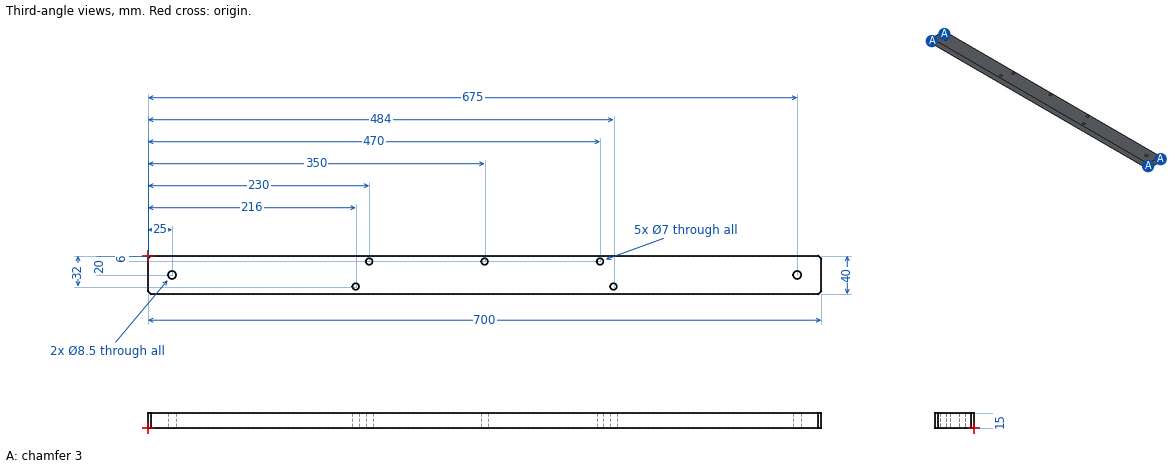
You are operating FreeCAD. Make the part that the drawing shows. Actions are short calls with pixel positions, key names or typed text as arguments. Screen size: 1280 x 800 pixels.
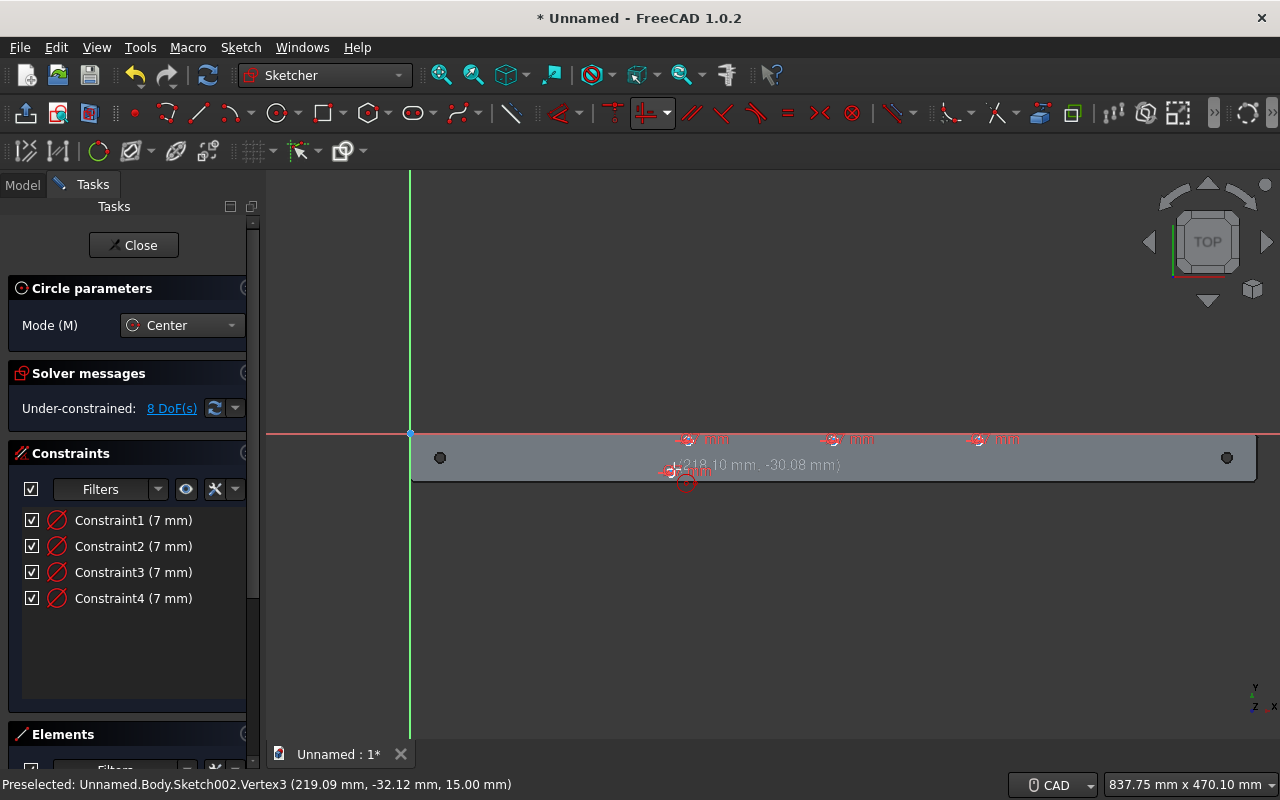
scroll(996, 472, up, 9)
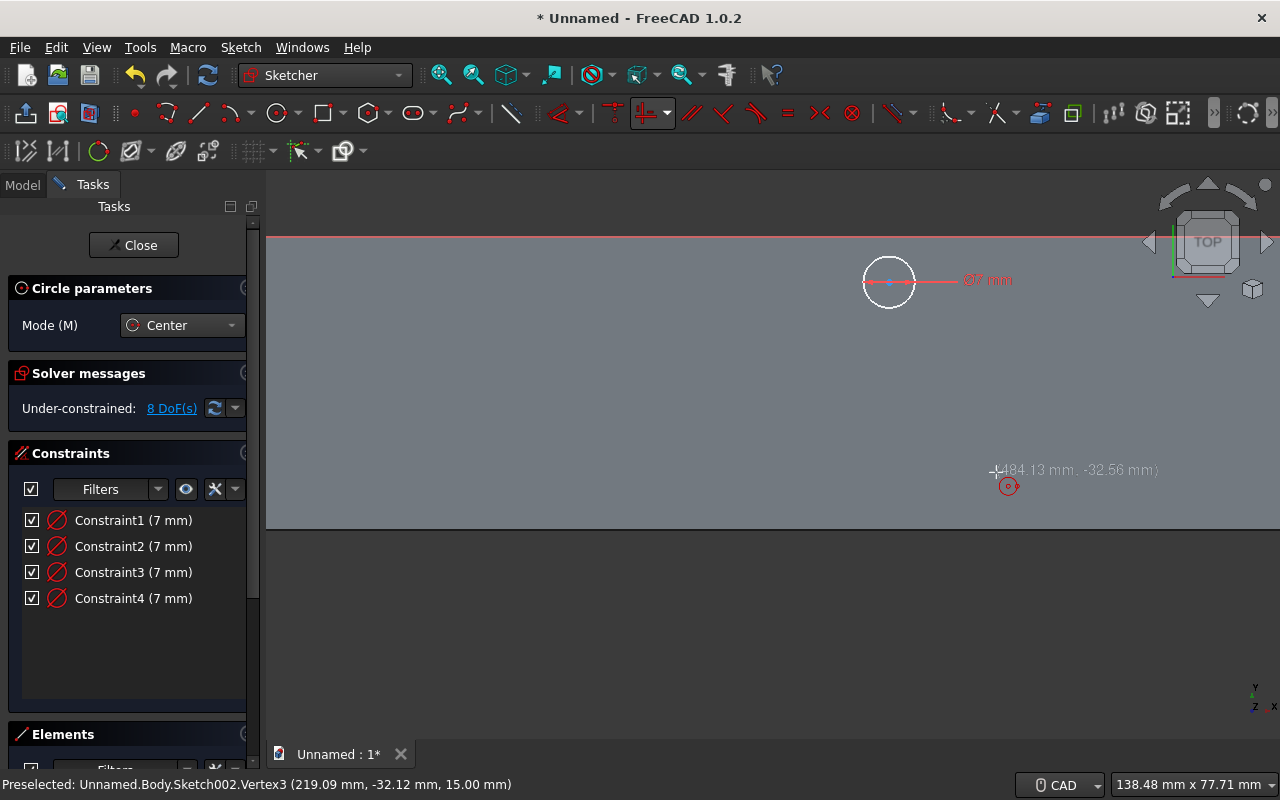
scroll(996, 472, down, 9)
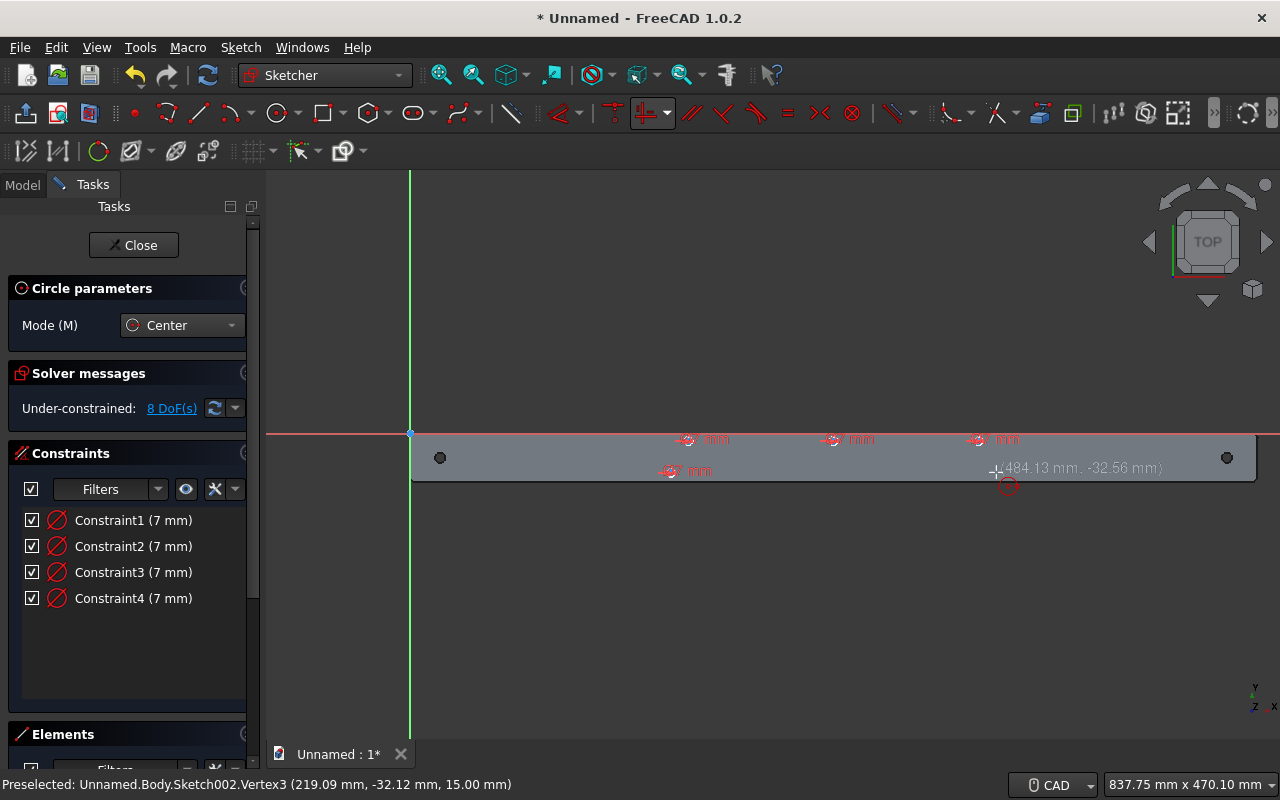
click(996, 472)
move(999, 469)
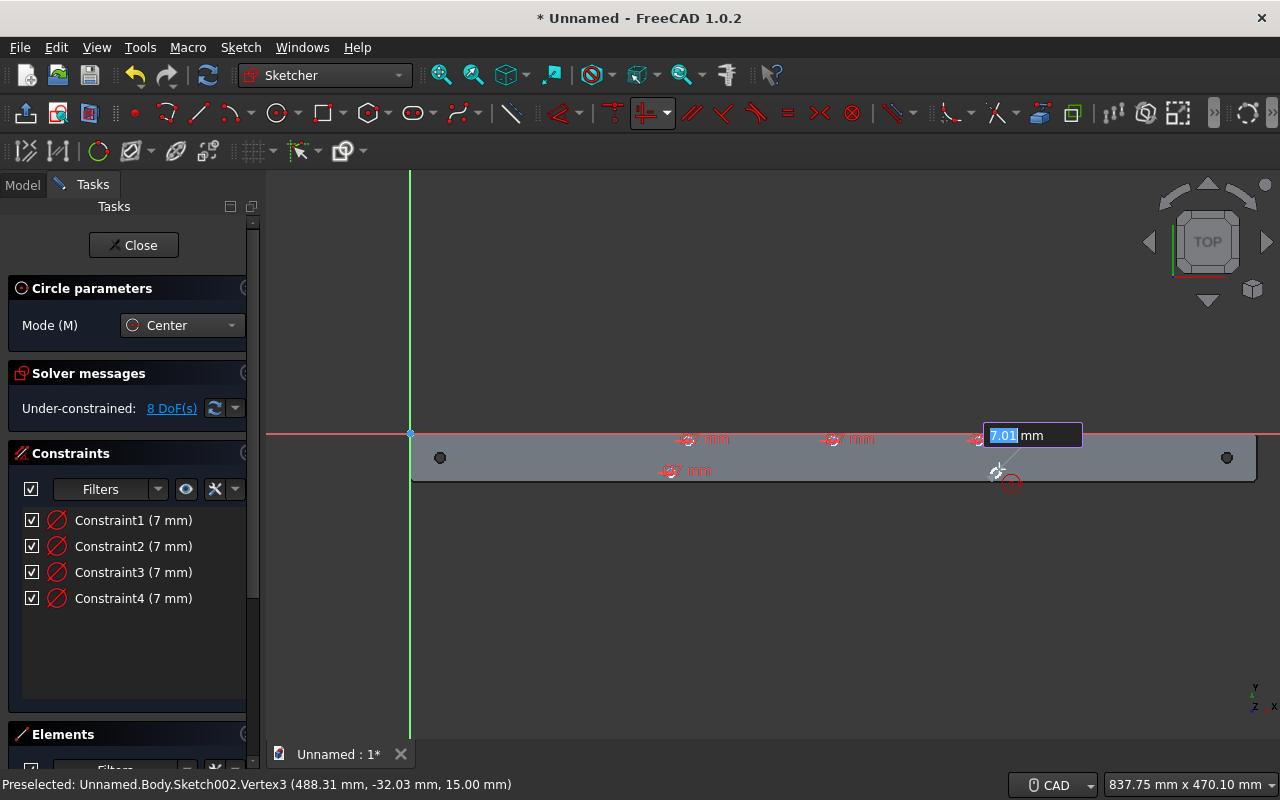
text(7)
key(Return)
key(Escape)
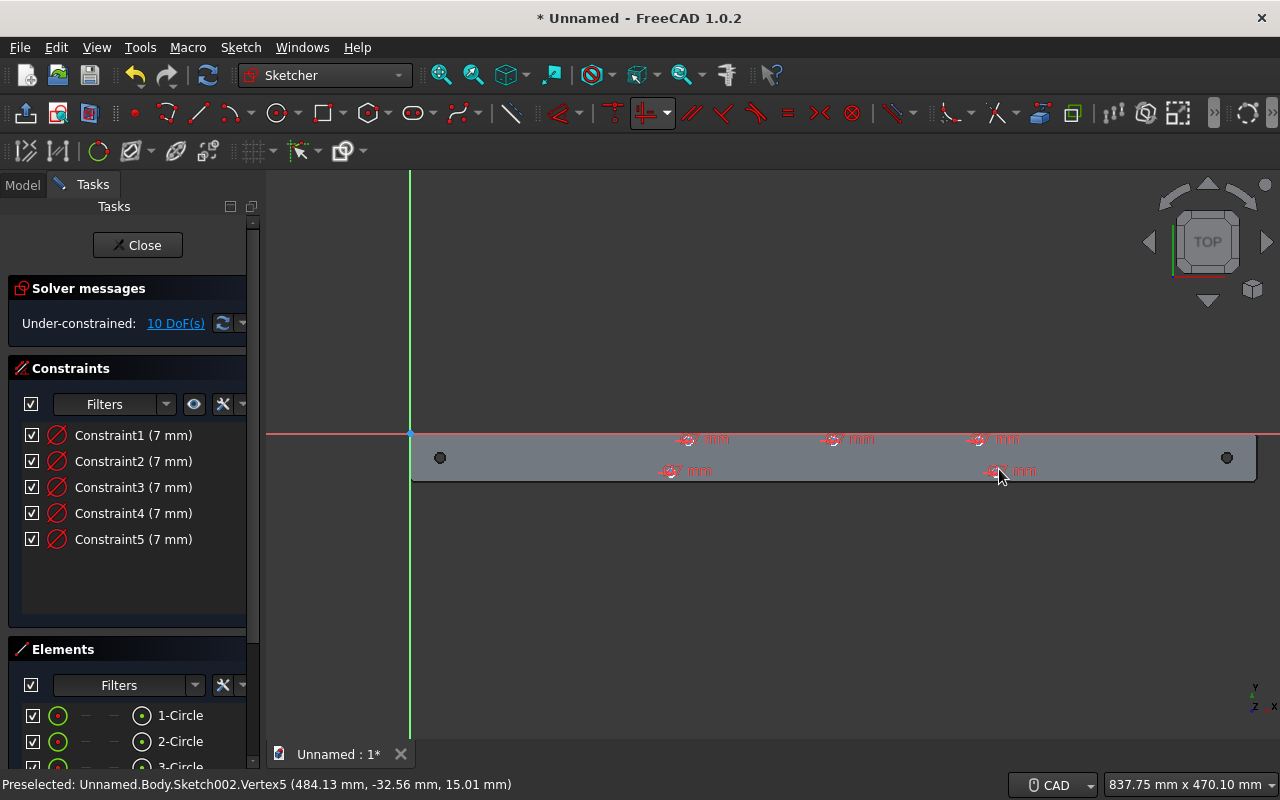
click(979, 441)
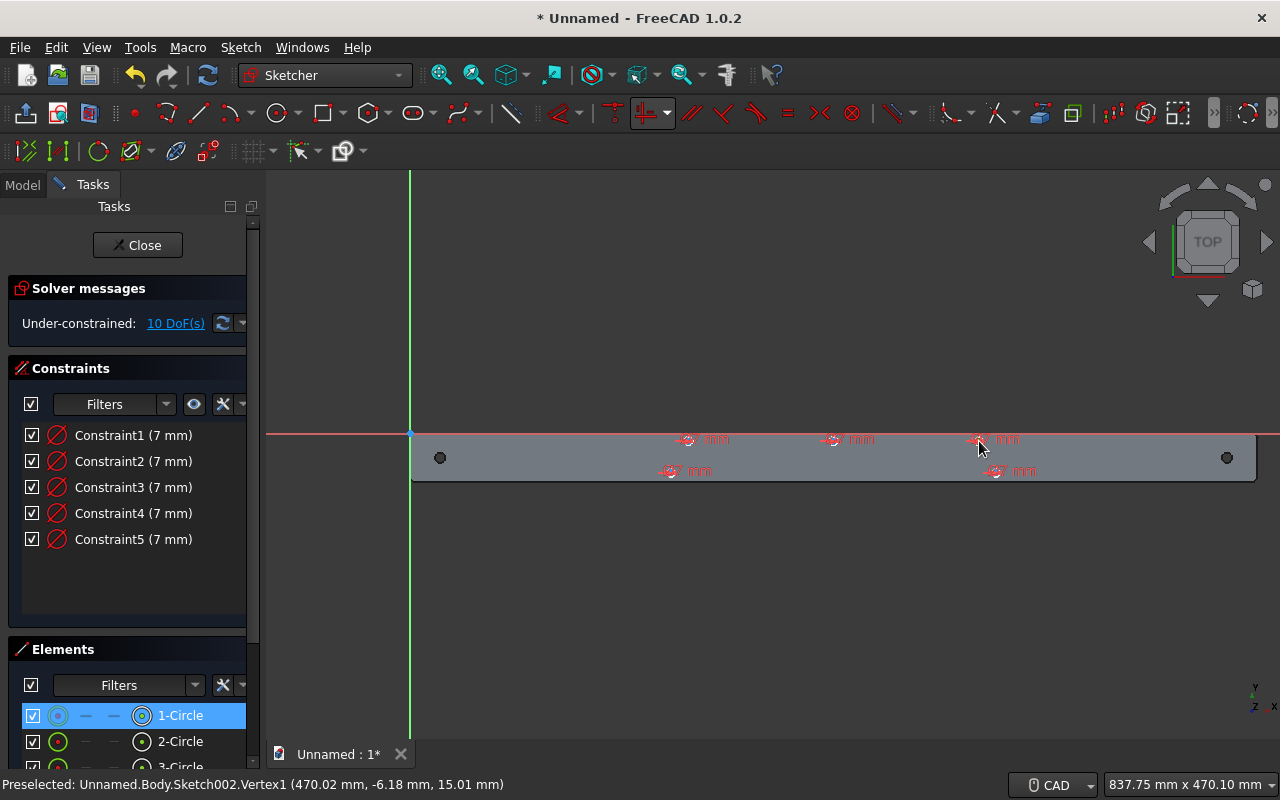
click(834, 441)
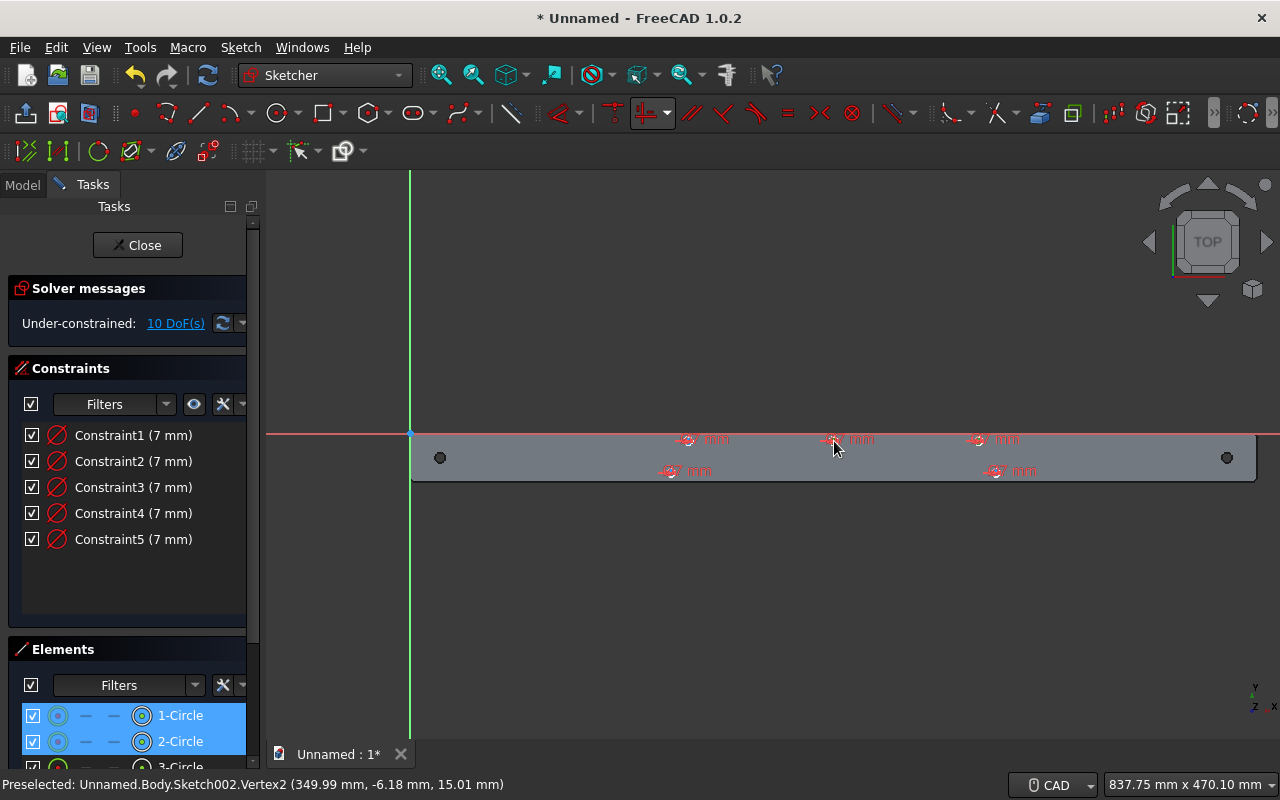
click(670, 114)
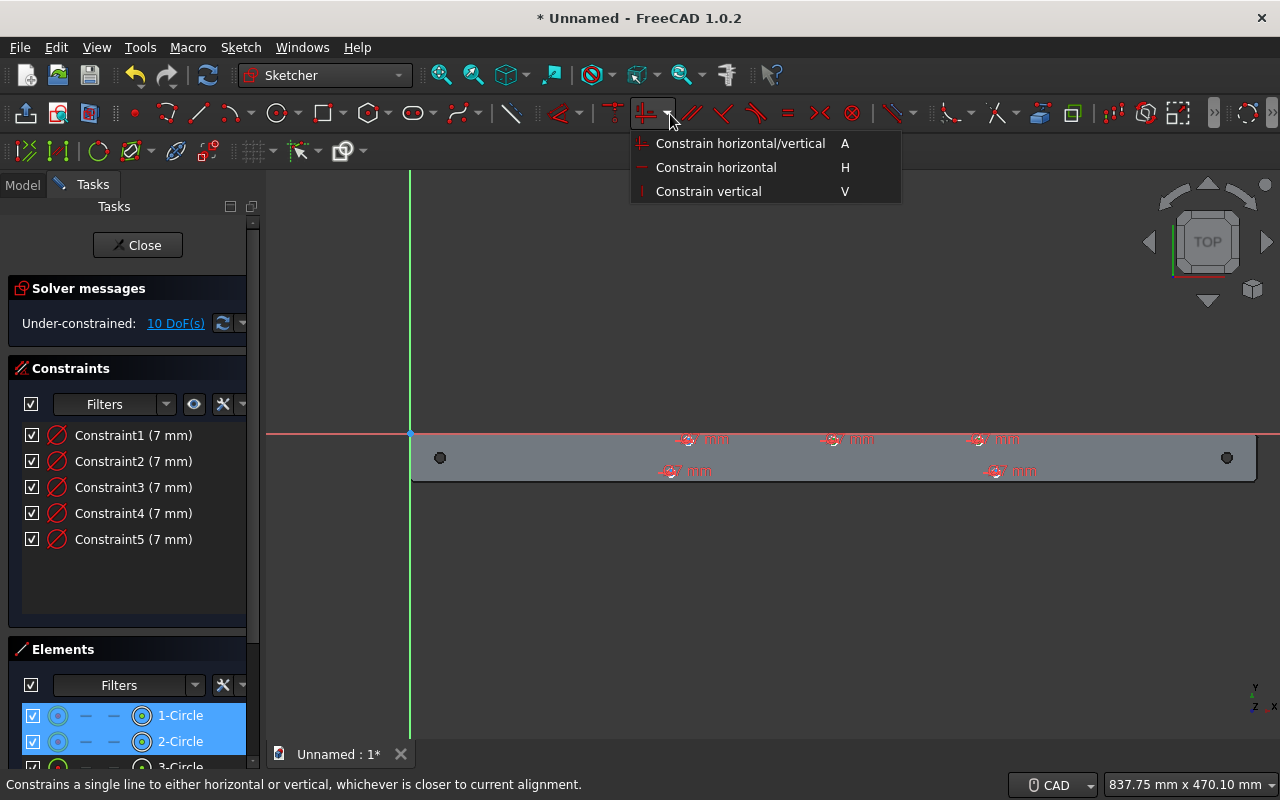
click(766, 167)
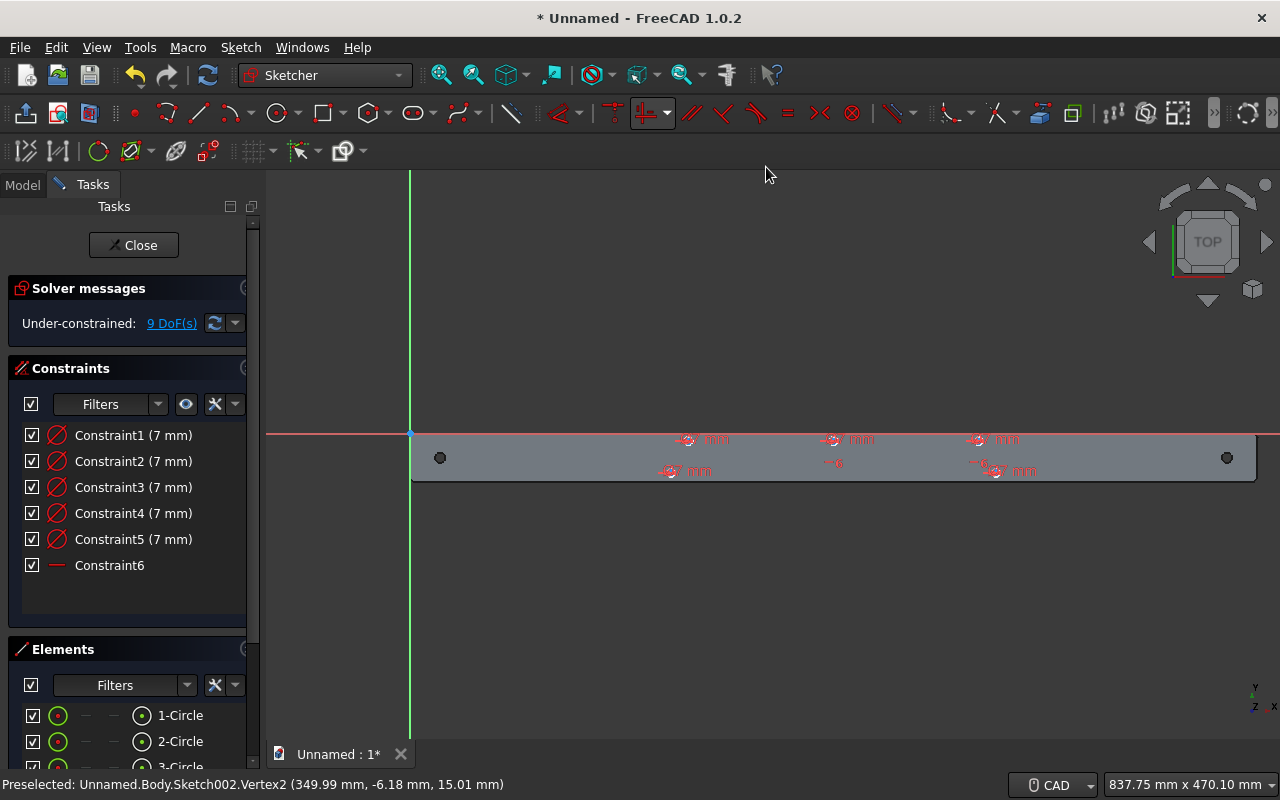
click(834, 441)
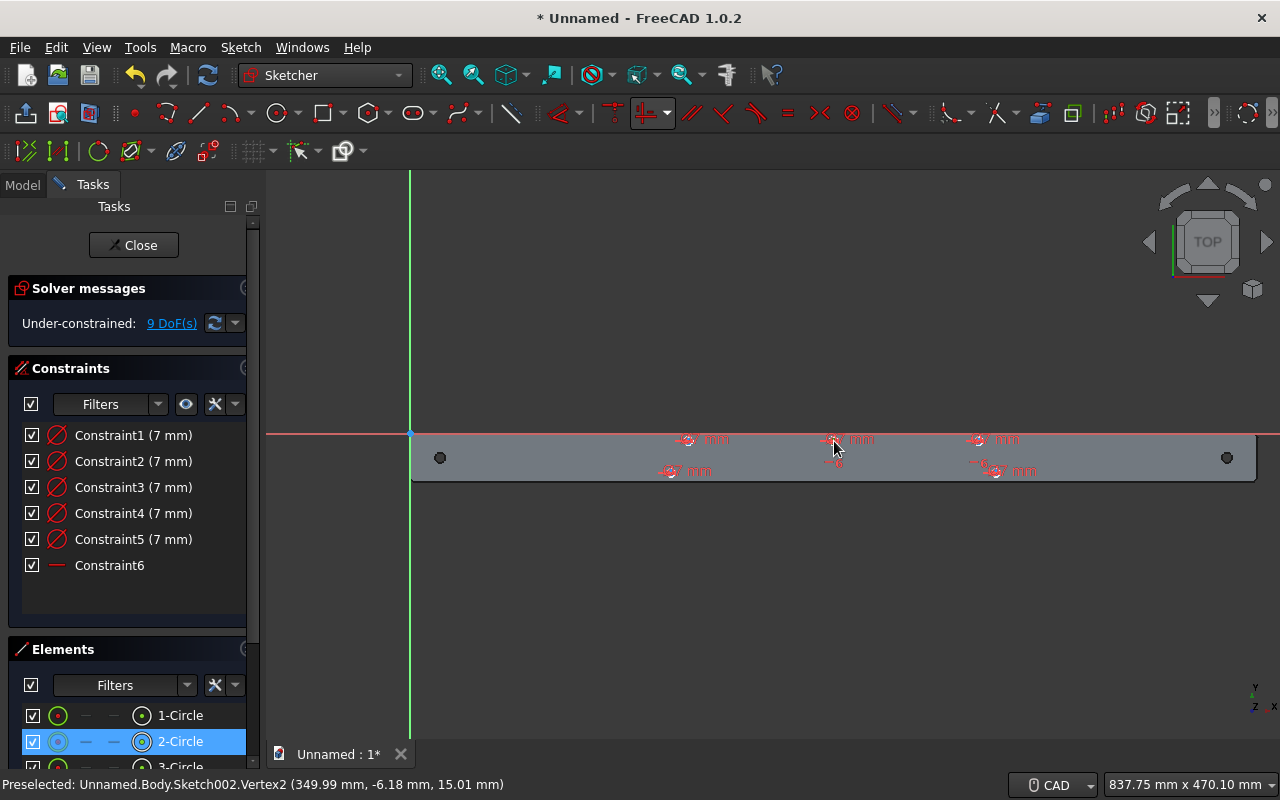
click(688, 441)